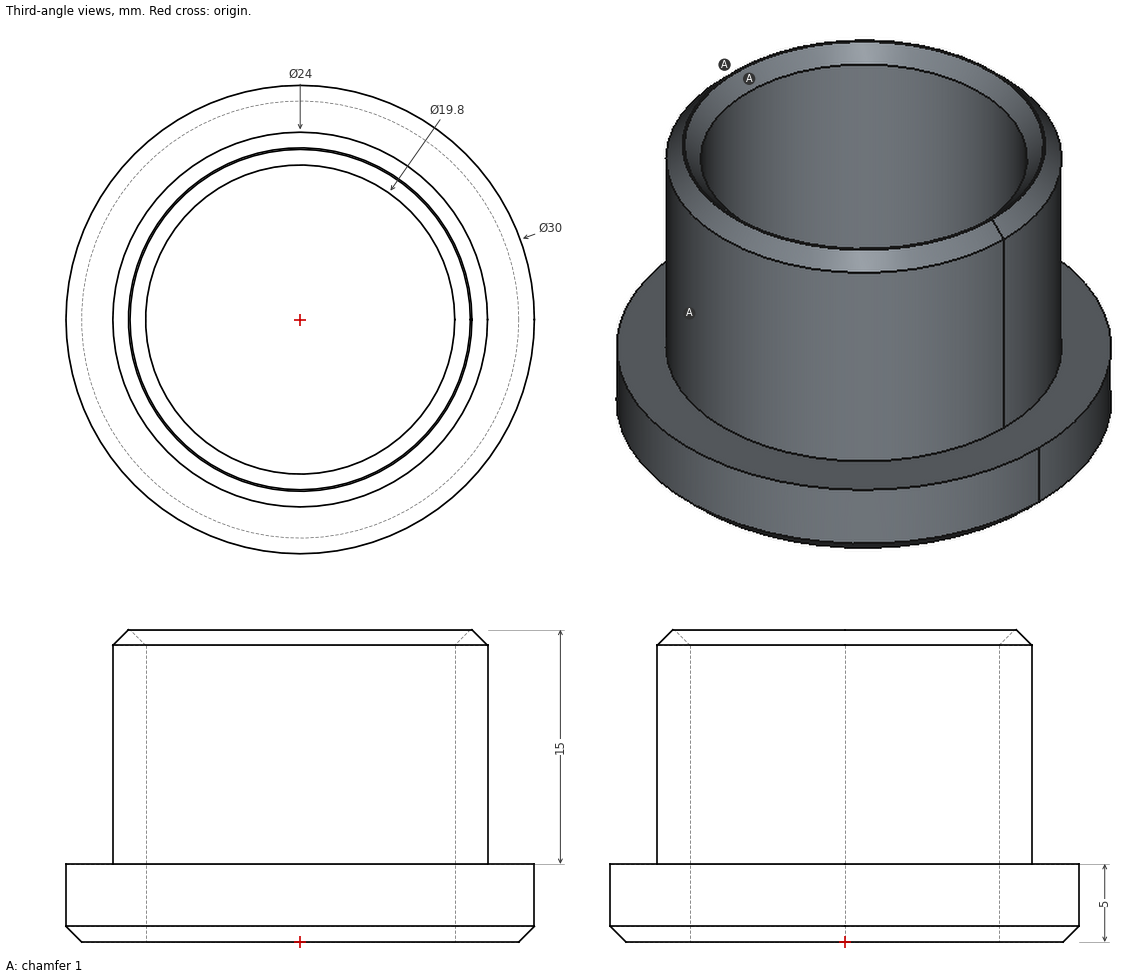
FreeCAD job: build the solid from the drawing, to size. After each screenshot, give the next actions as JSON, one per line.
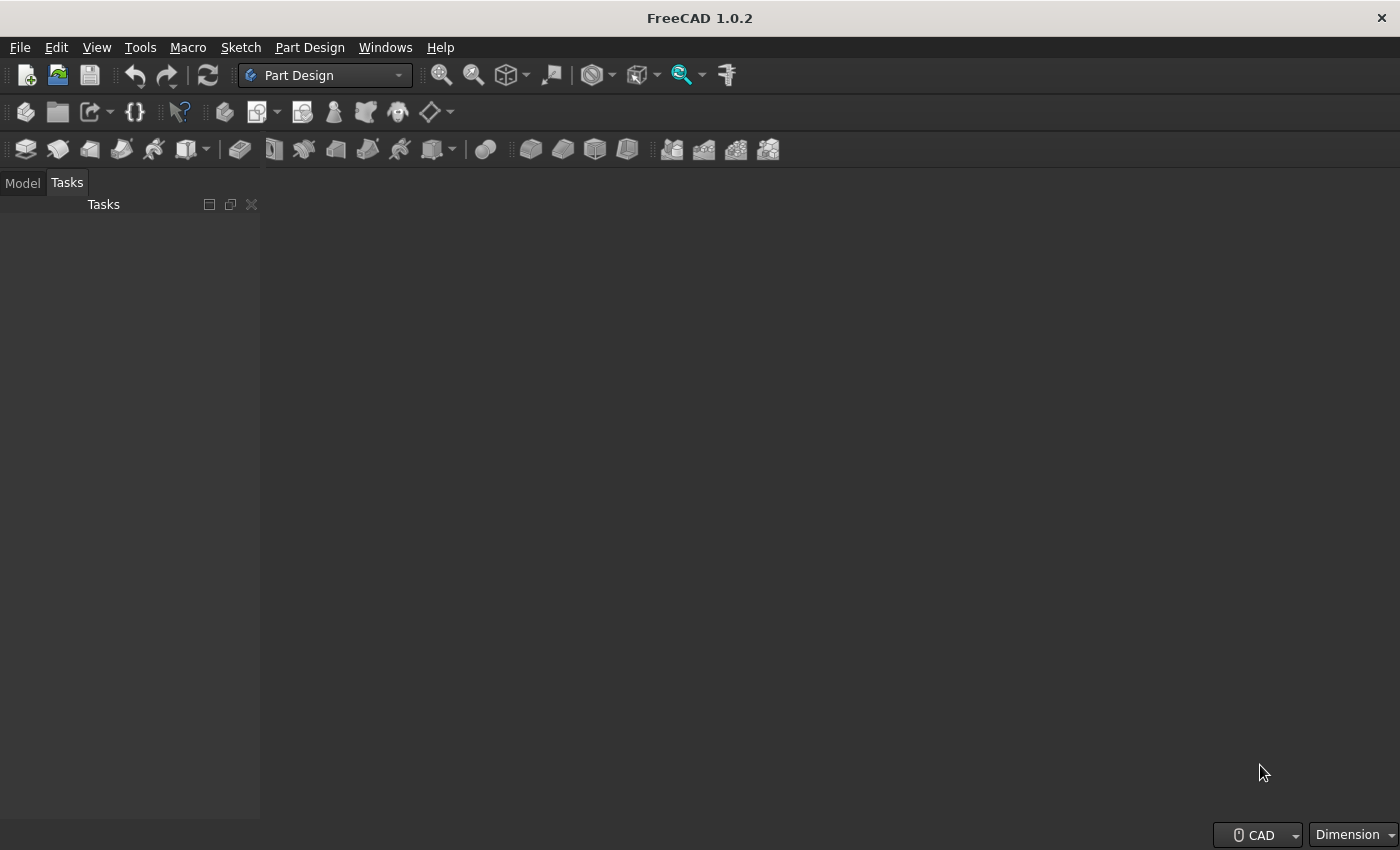
{"action": "key", "text": "ctrl+n"}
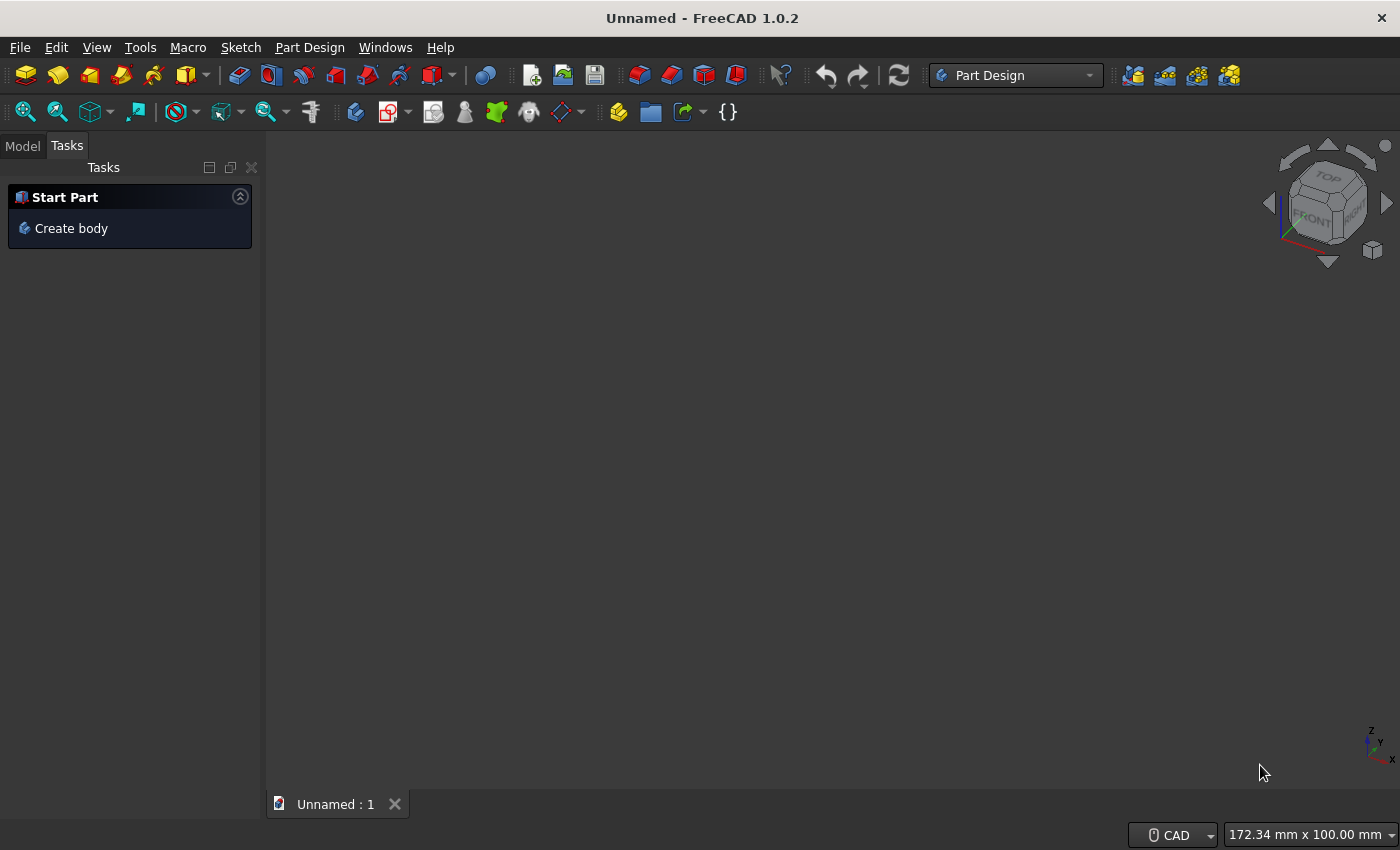
{"action": "left_click", "coordinate": [388, 112]}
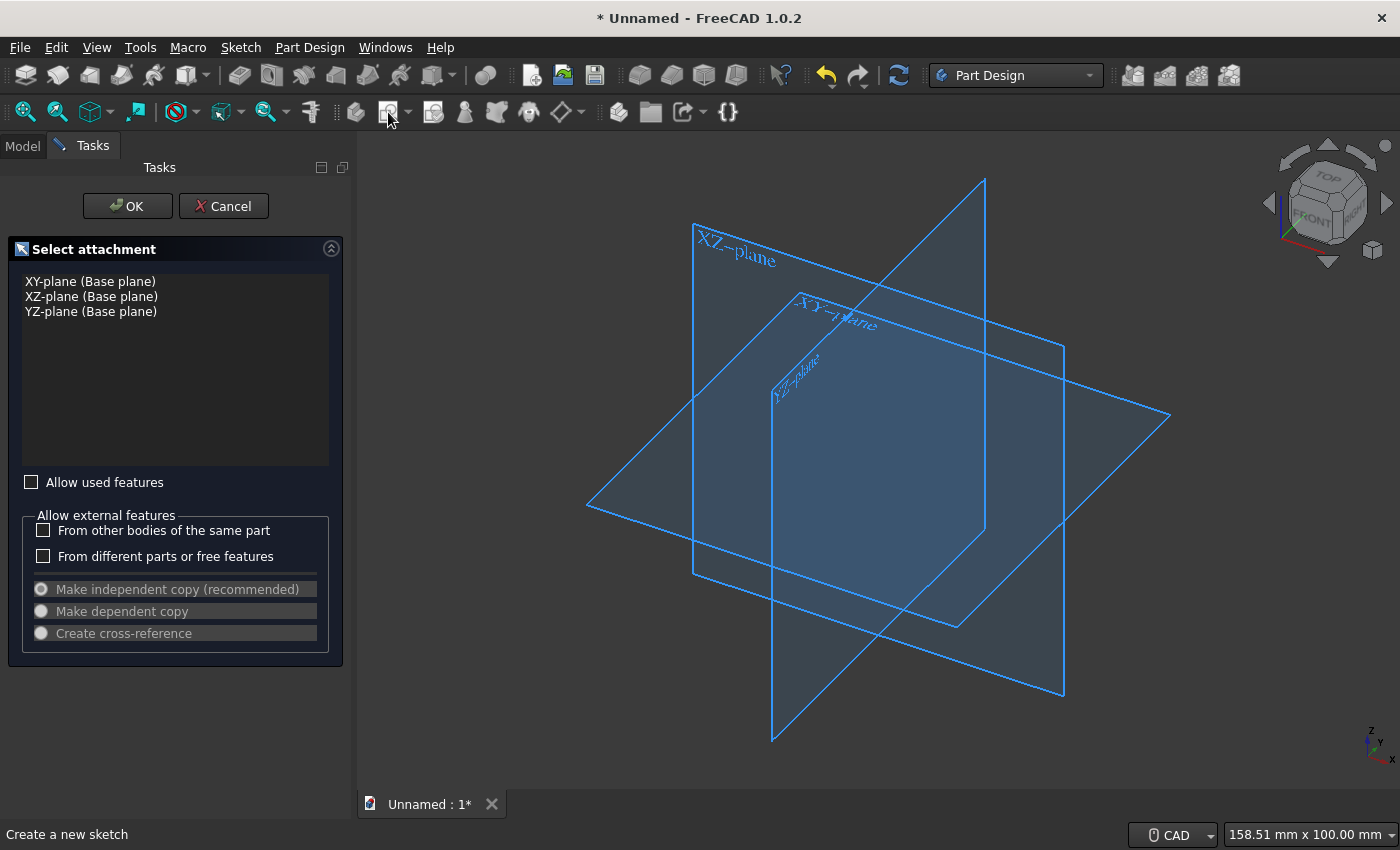
{"action": "left_click", "coordinate": [82, 282]}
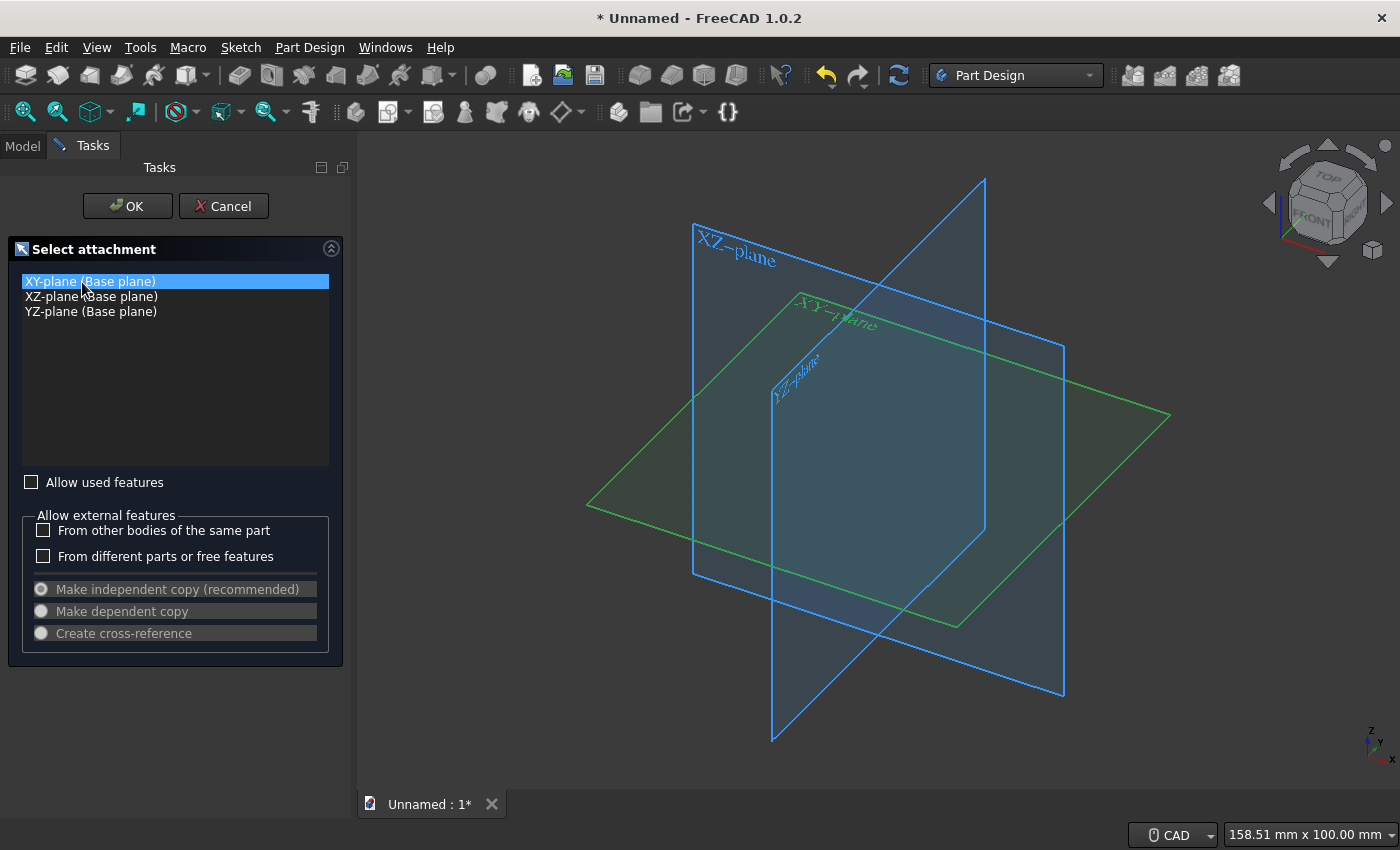
{"action": "left_click", "coordinate": [128, 206]}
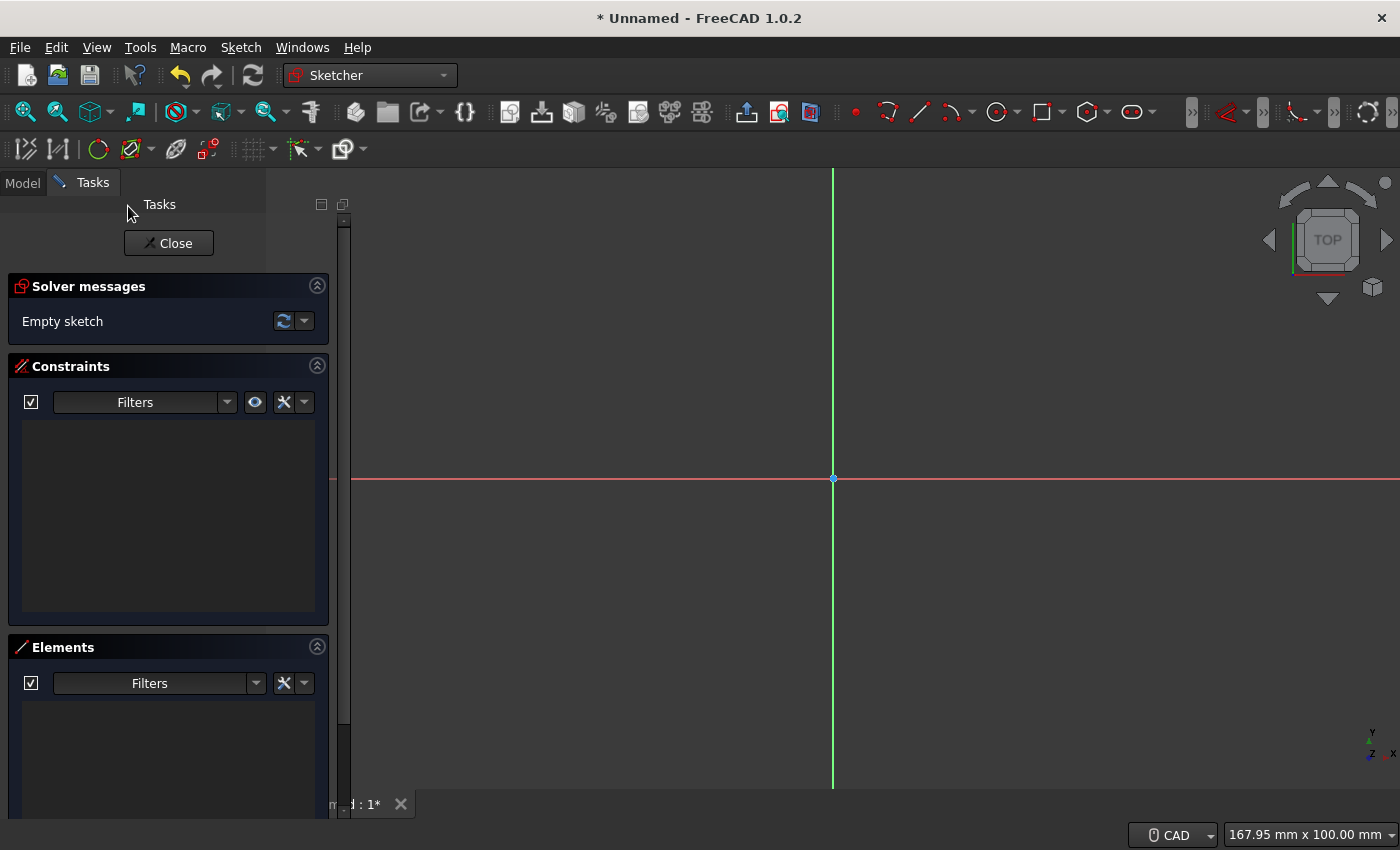
{"action": "scroll", "coordinate": [889, 478], "scroll_direction": "up", "scroll_amount": 4}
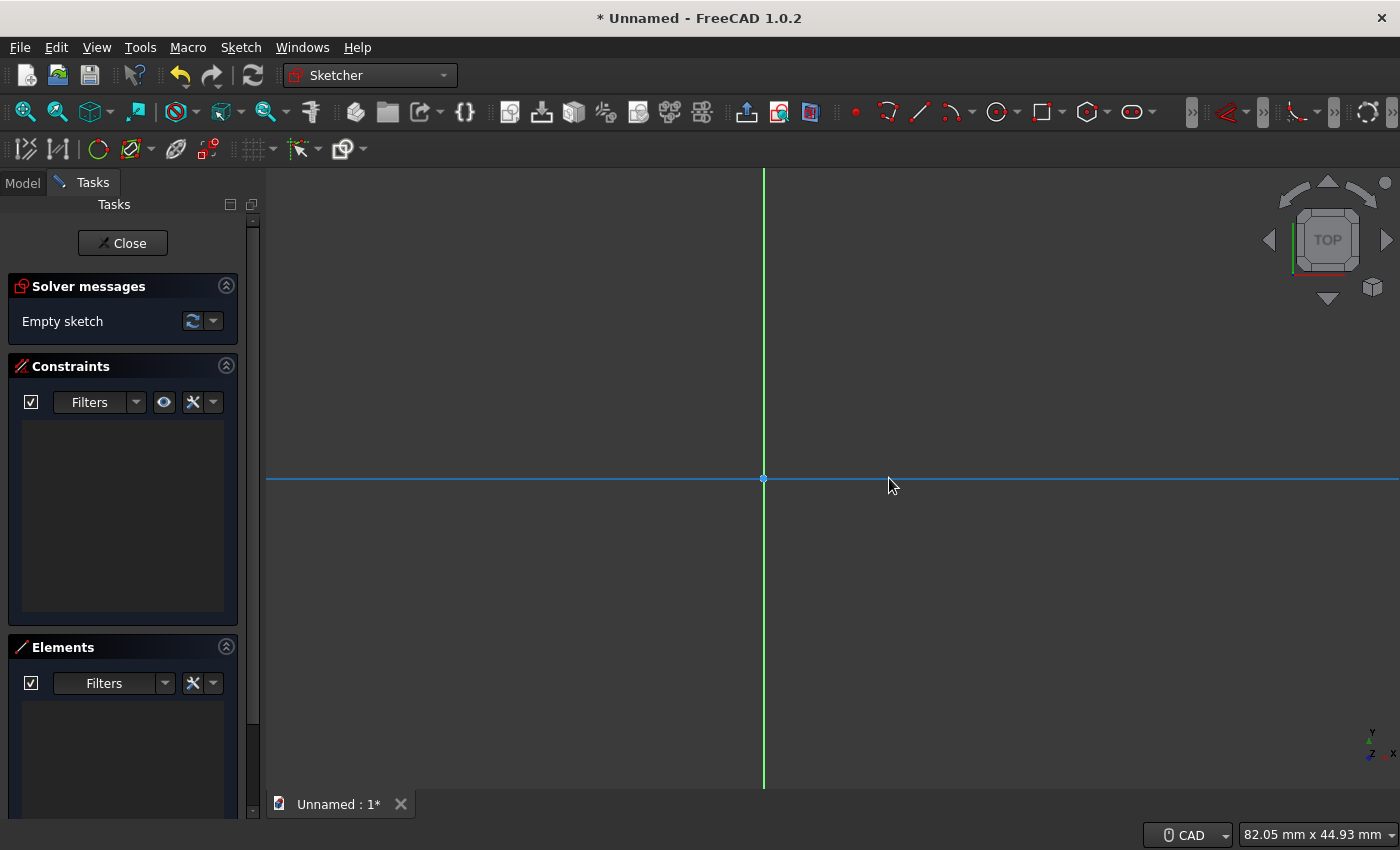
{"action": "left_click", "coordinate": [998, 112]}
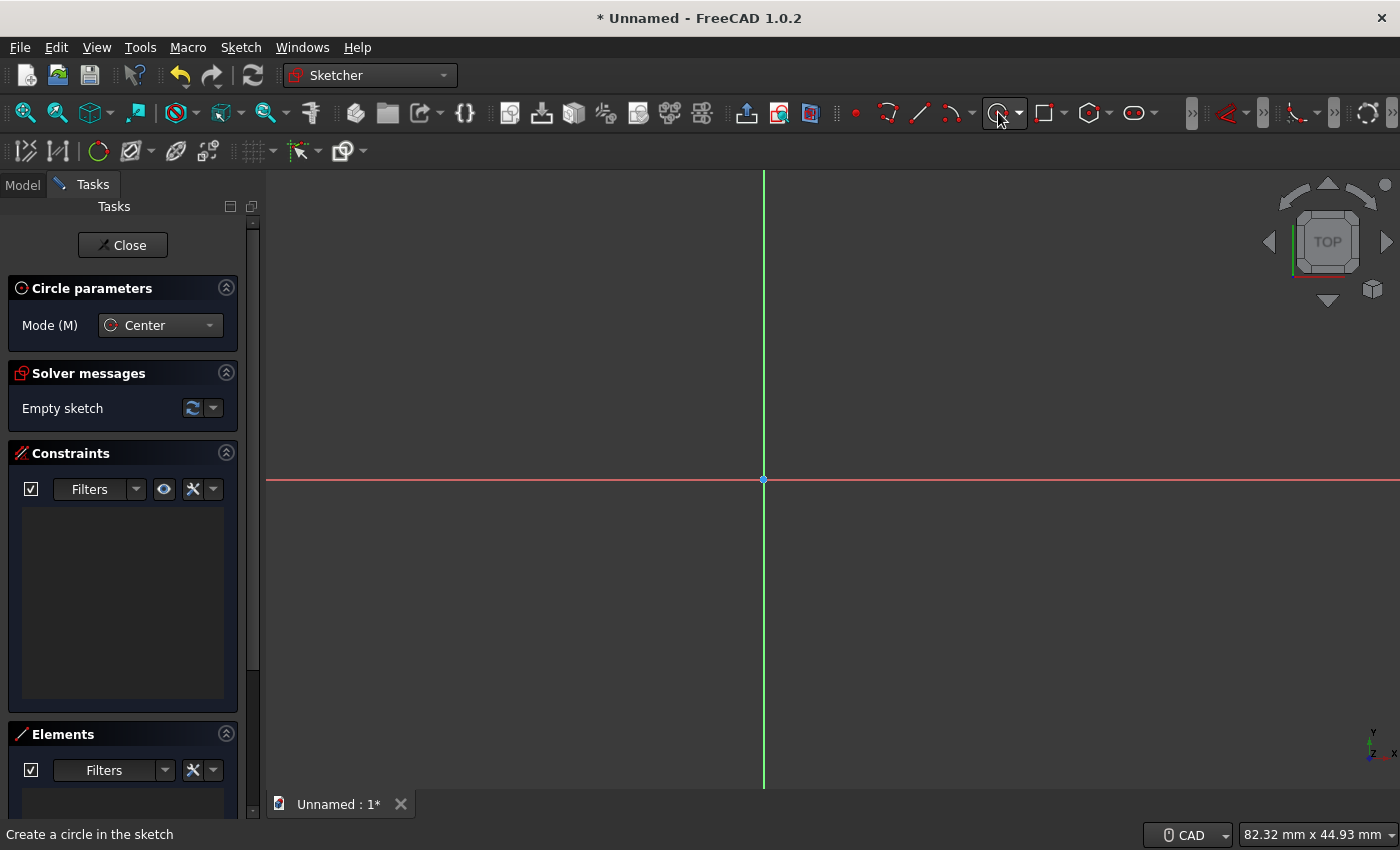
{"action": "left_click", "coordinate": [764, 480]}
{"action": "mouse_move", "coordinate": [910, 333]}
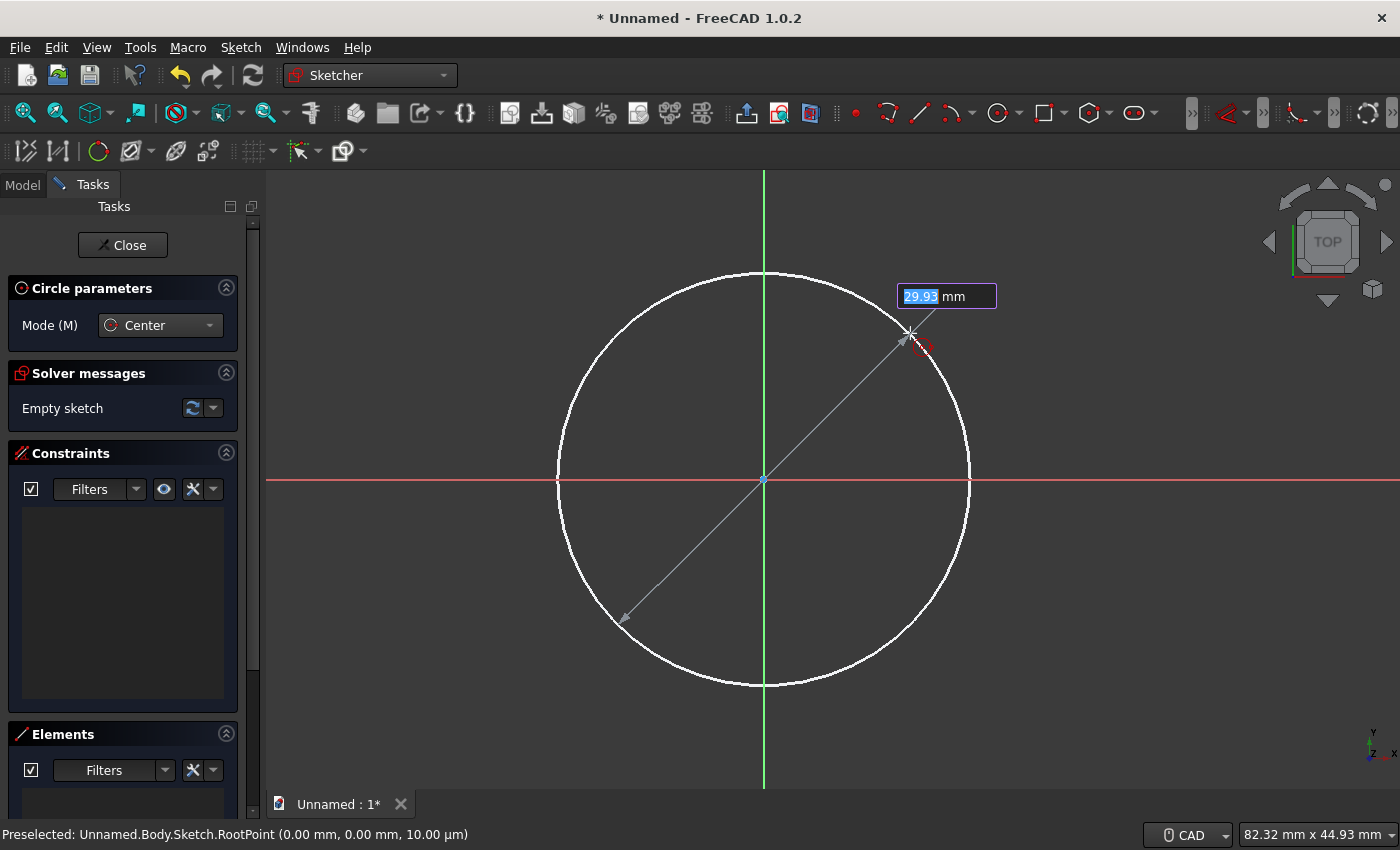
{"action": "type", "text": "30"}
{"action": "key", "text": "Return"}